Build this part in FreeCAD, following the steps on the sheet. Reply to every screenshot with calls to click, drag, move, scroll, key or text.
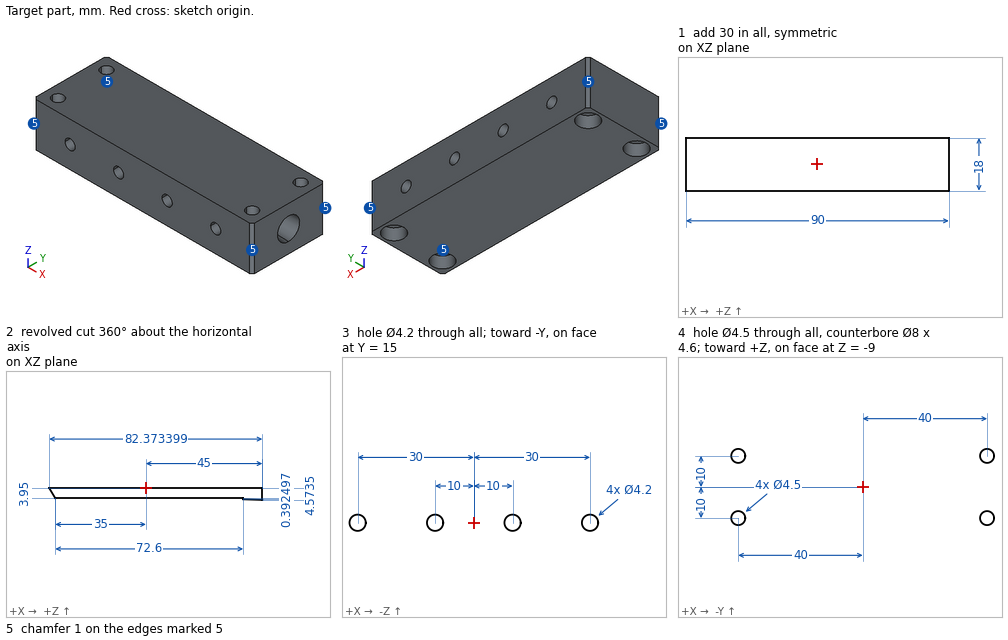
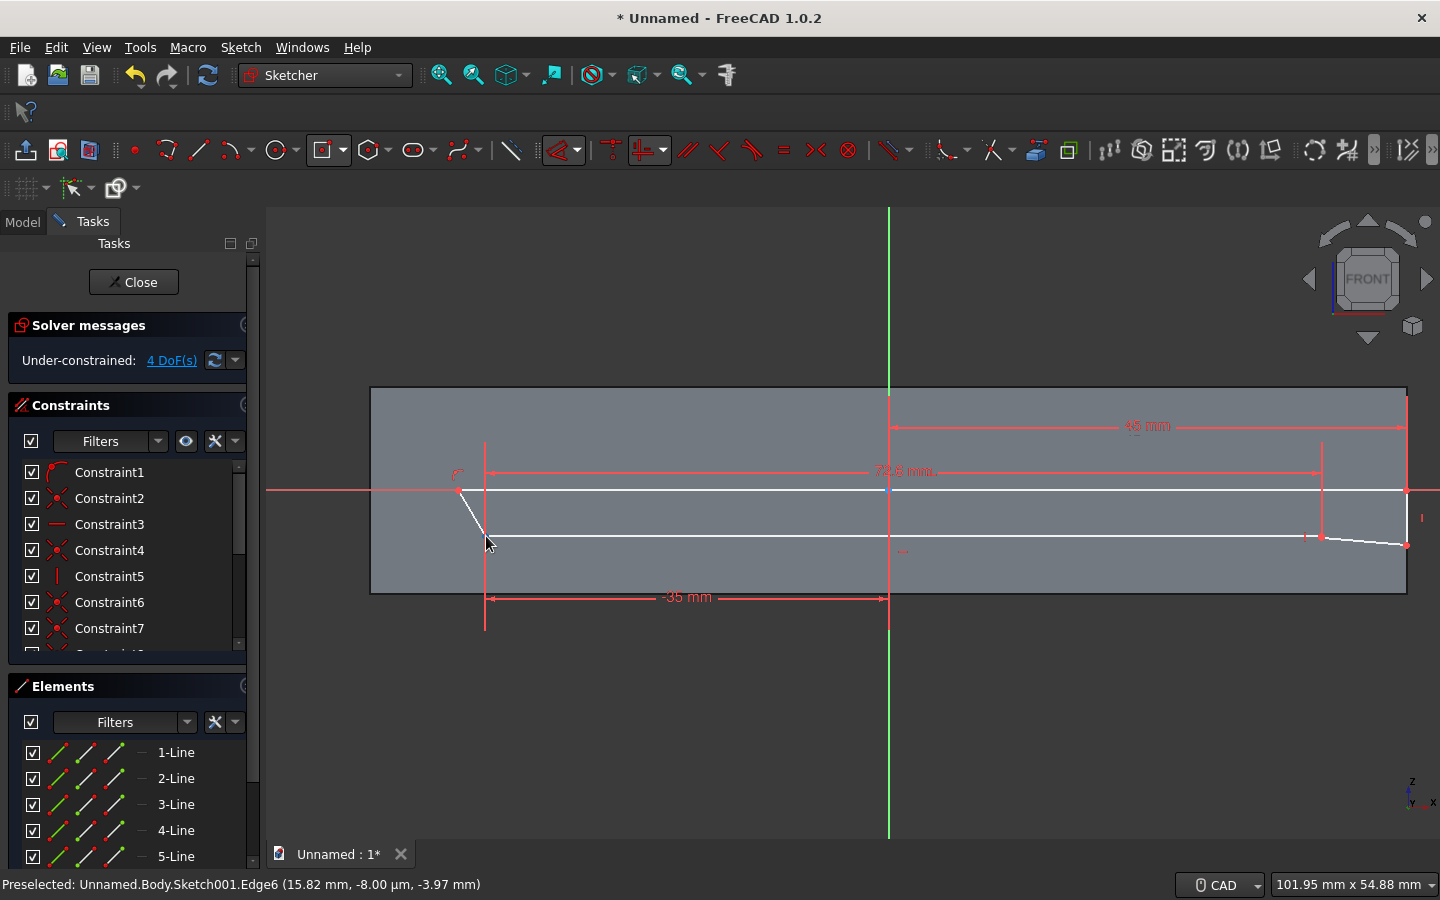
click(485, 536)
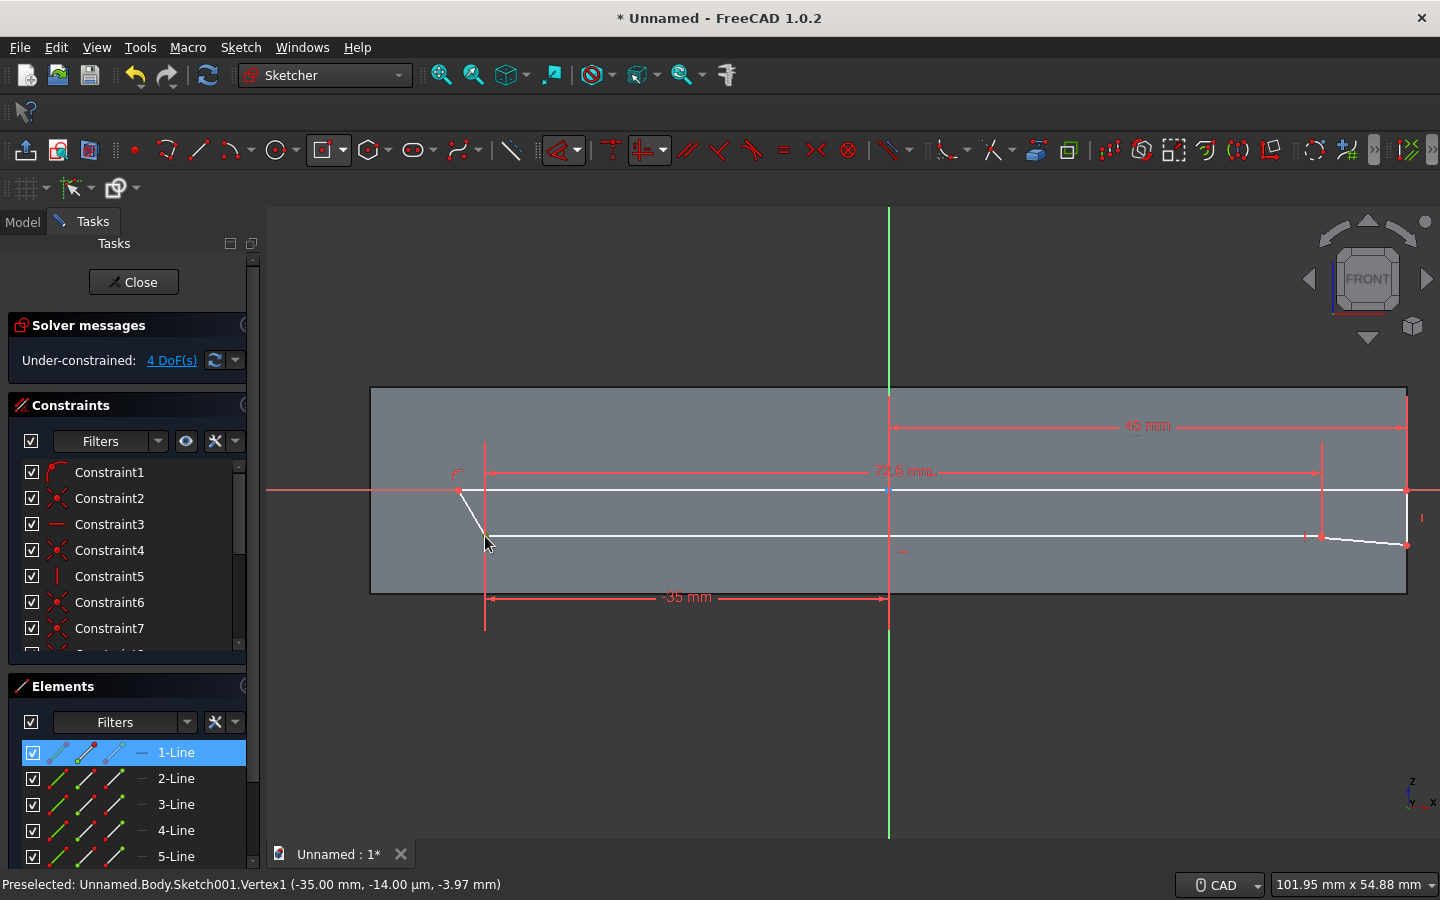
key(i)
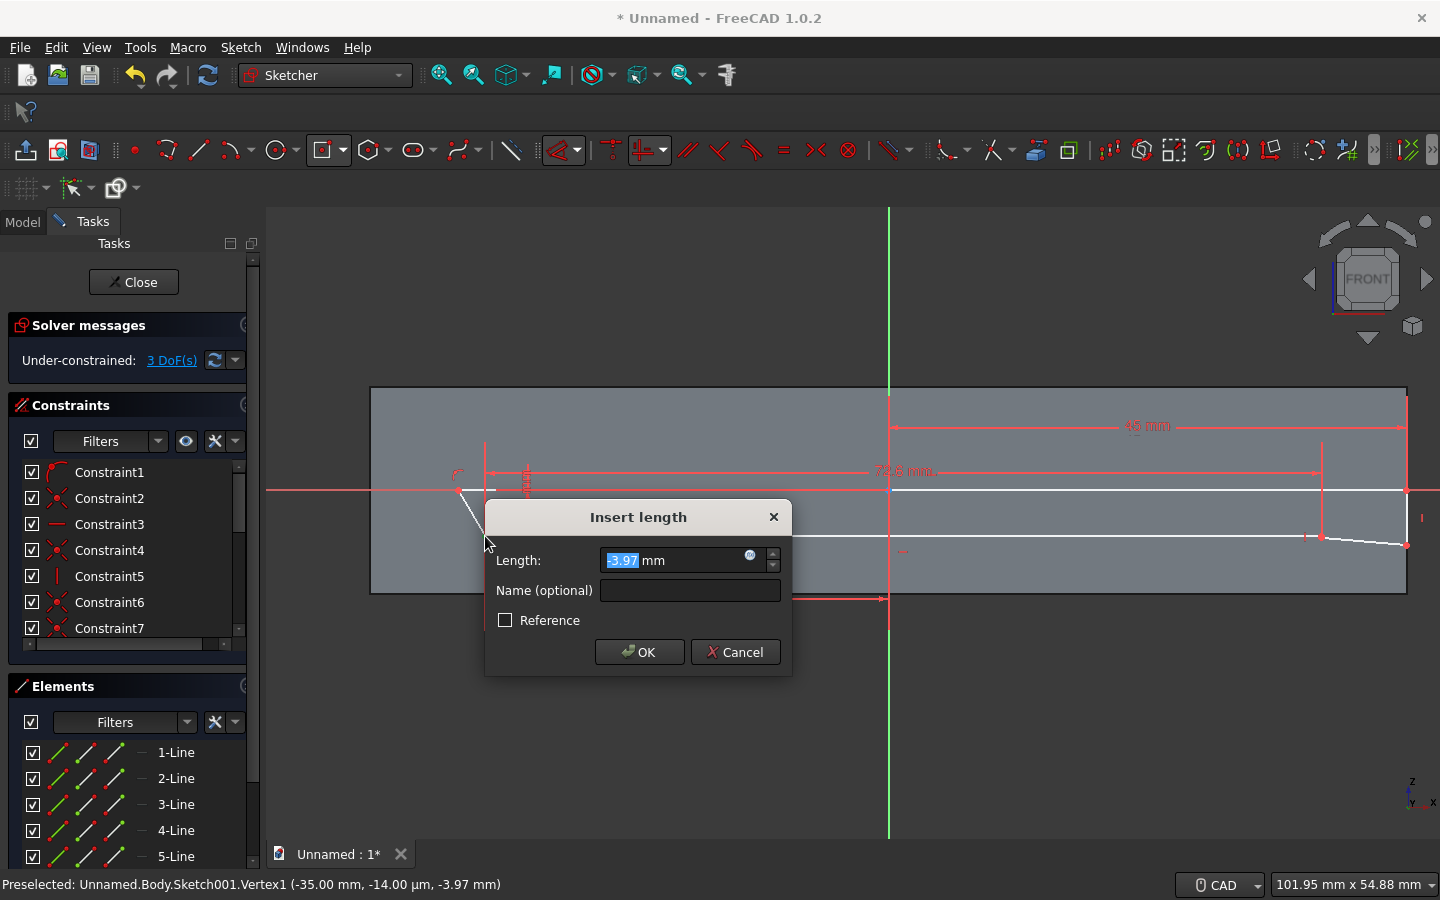
text(-3.95)
key(Return)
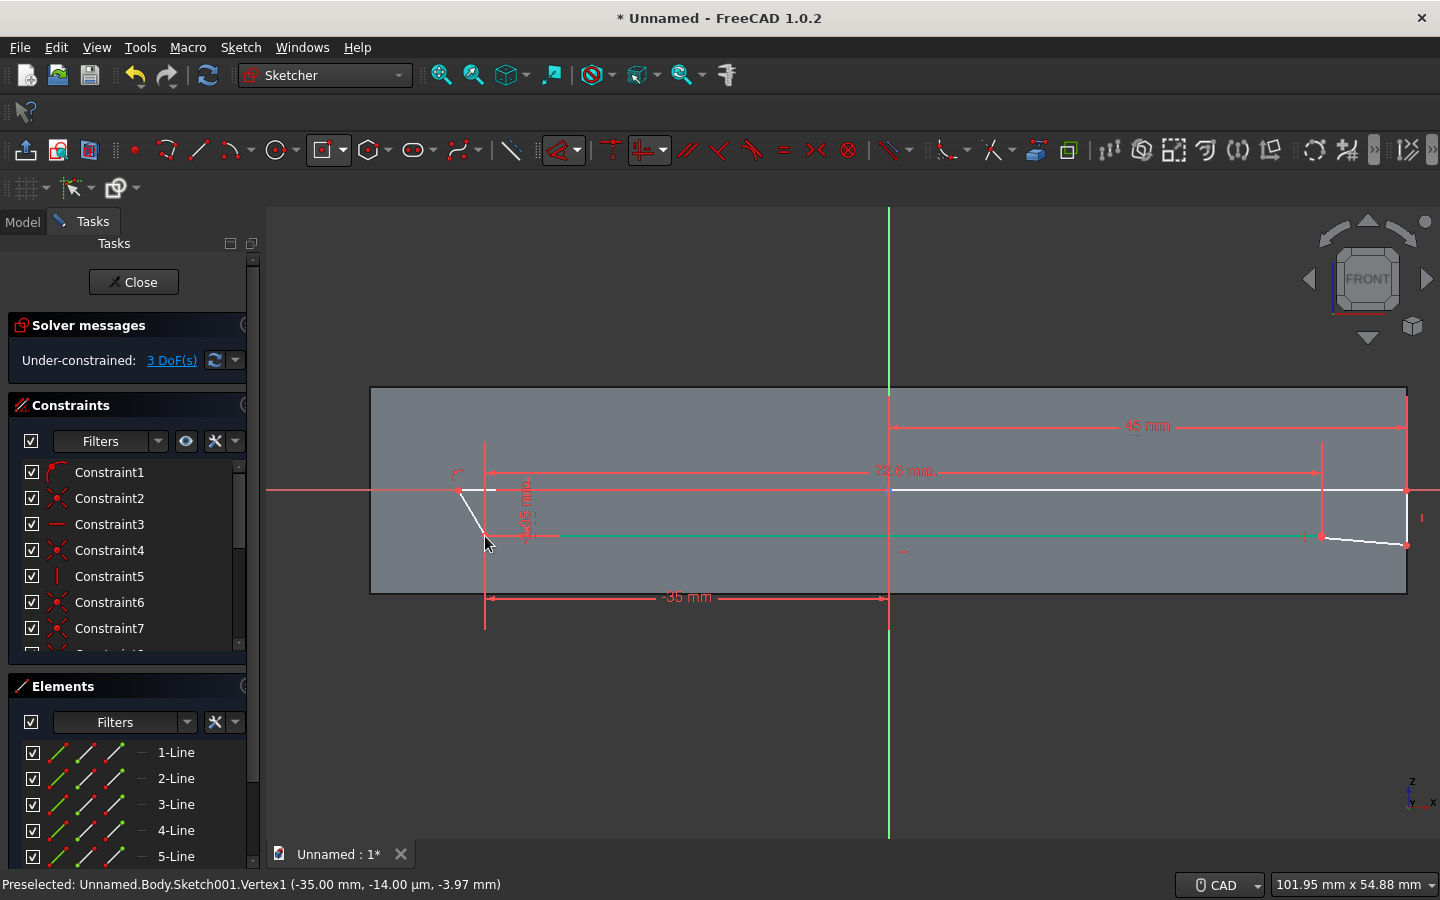
scroll(484, 536, down, 2)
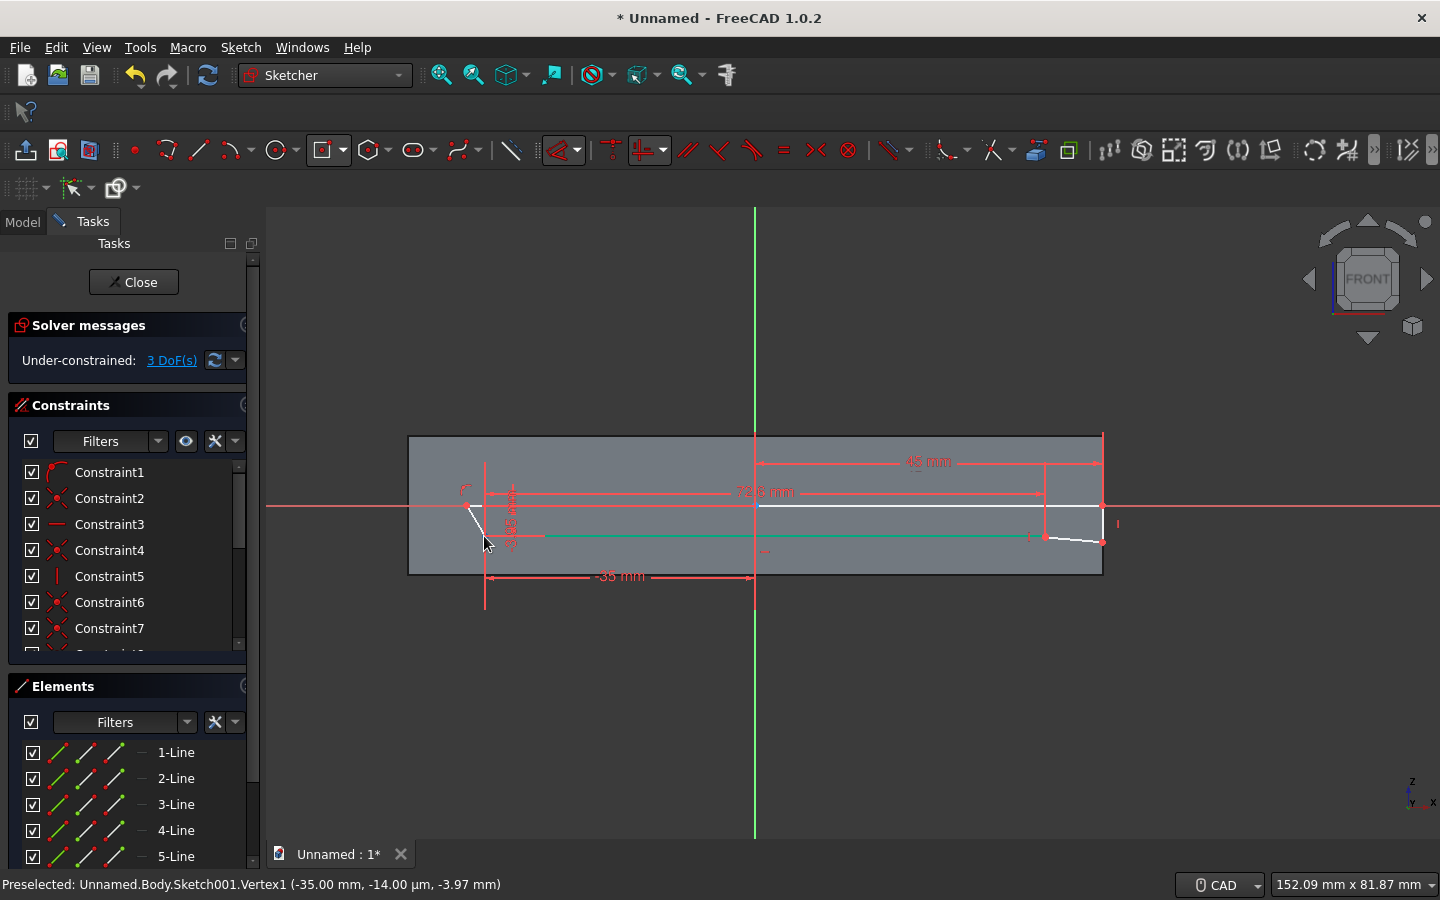
scroll(1103, 517, up, 2)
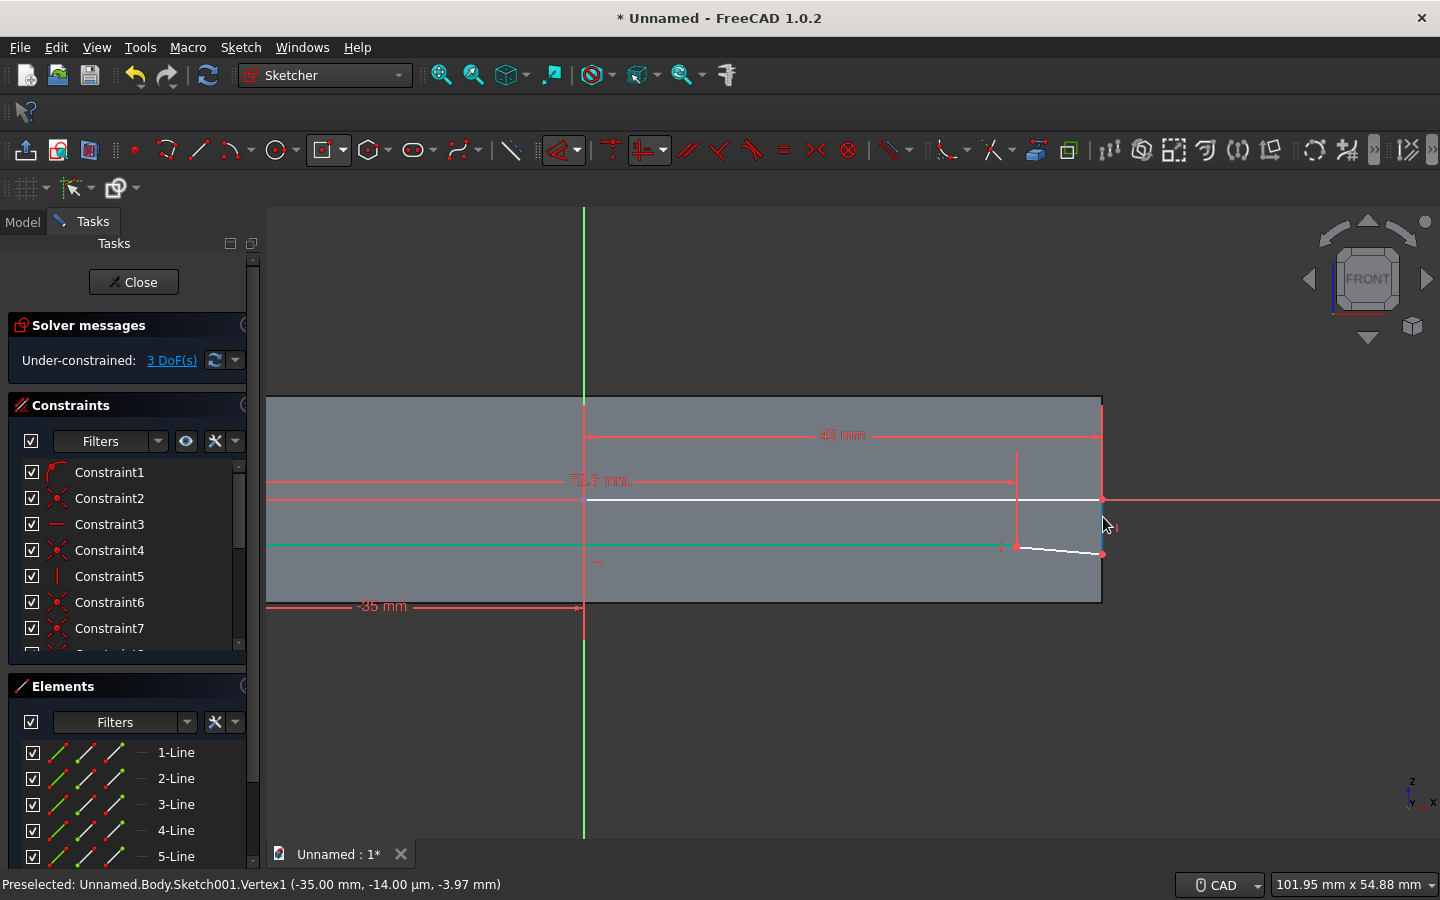
click(1102, 516)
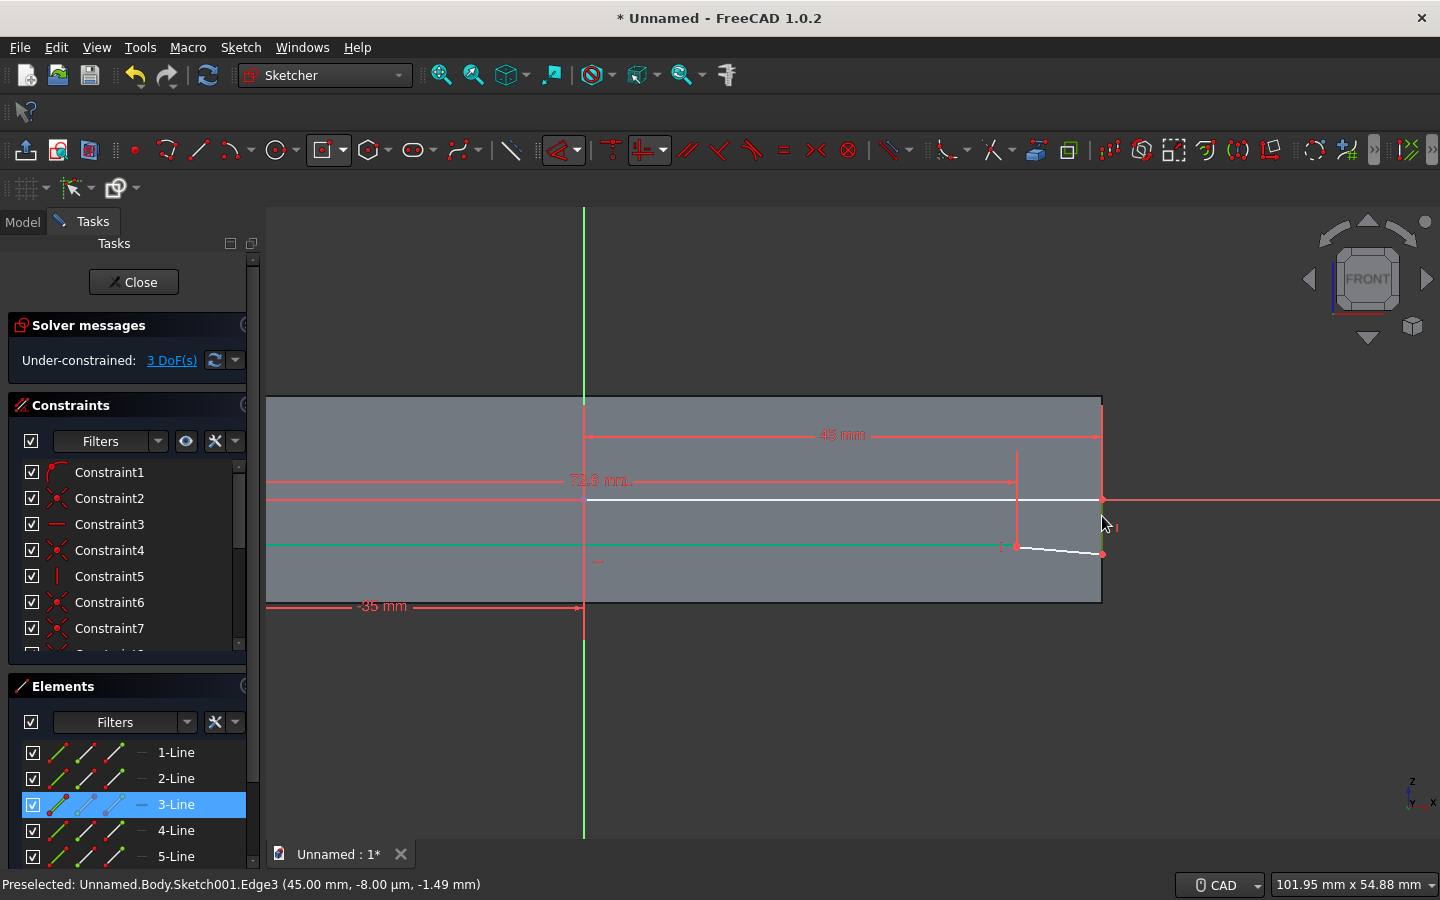
click(580, 150)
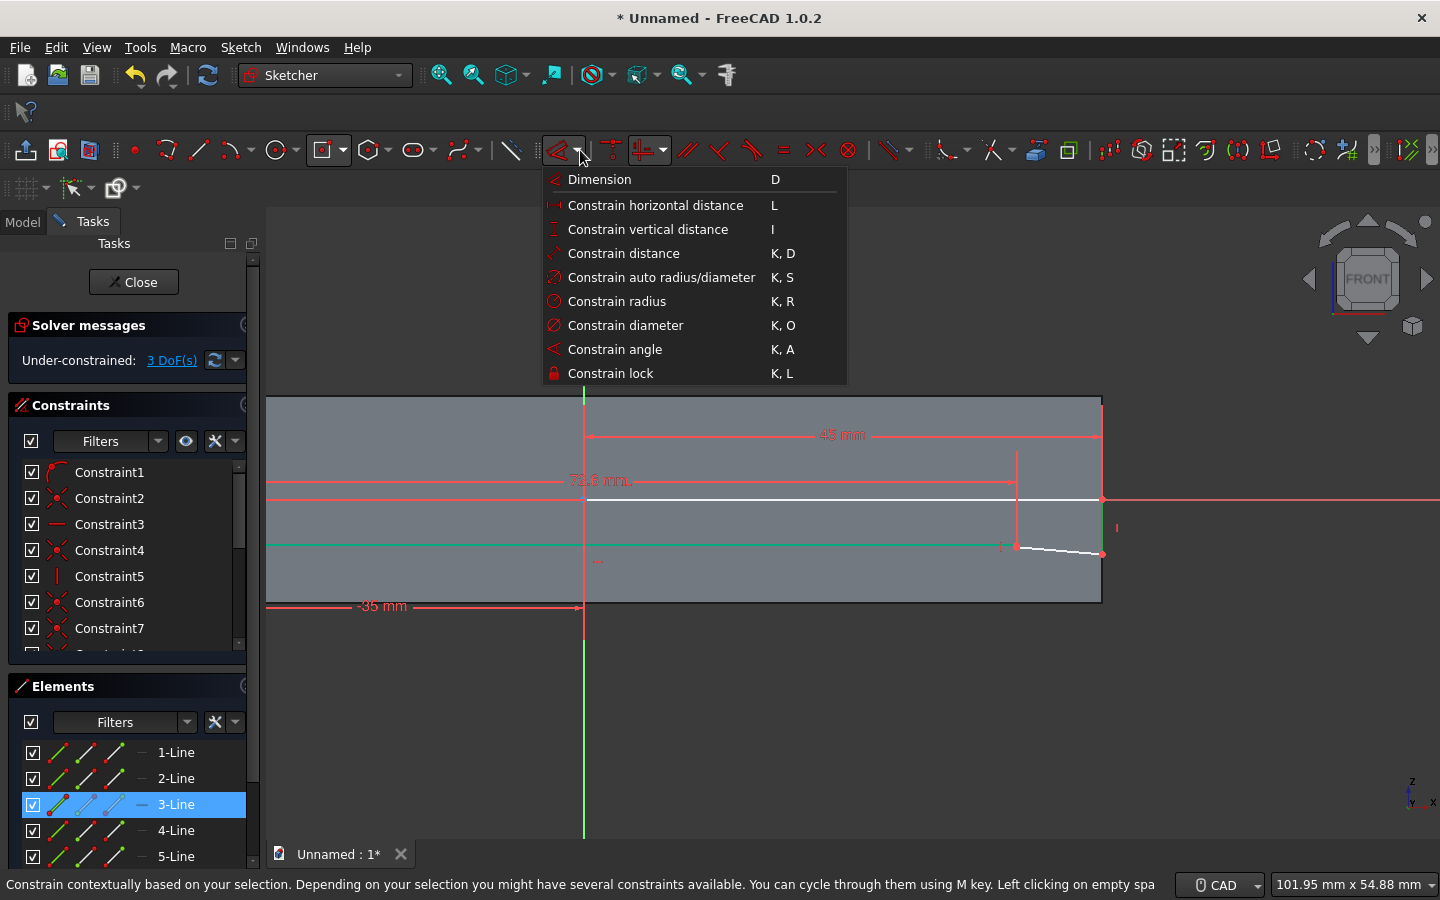
click(695, 229)